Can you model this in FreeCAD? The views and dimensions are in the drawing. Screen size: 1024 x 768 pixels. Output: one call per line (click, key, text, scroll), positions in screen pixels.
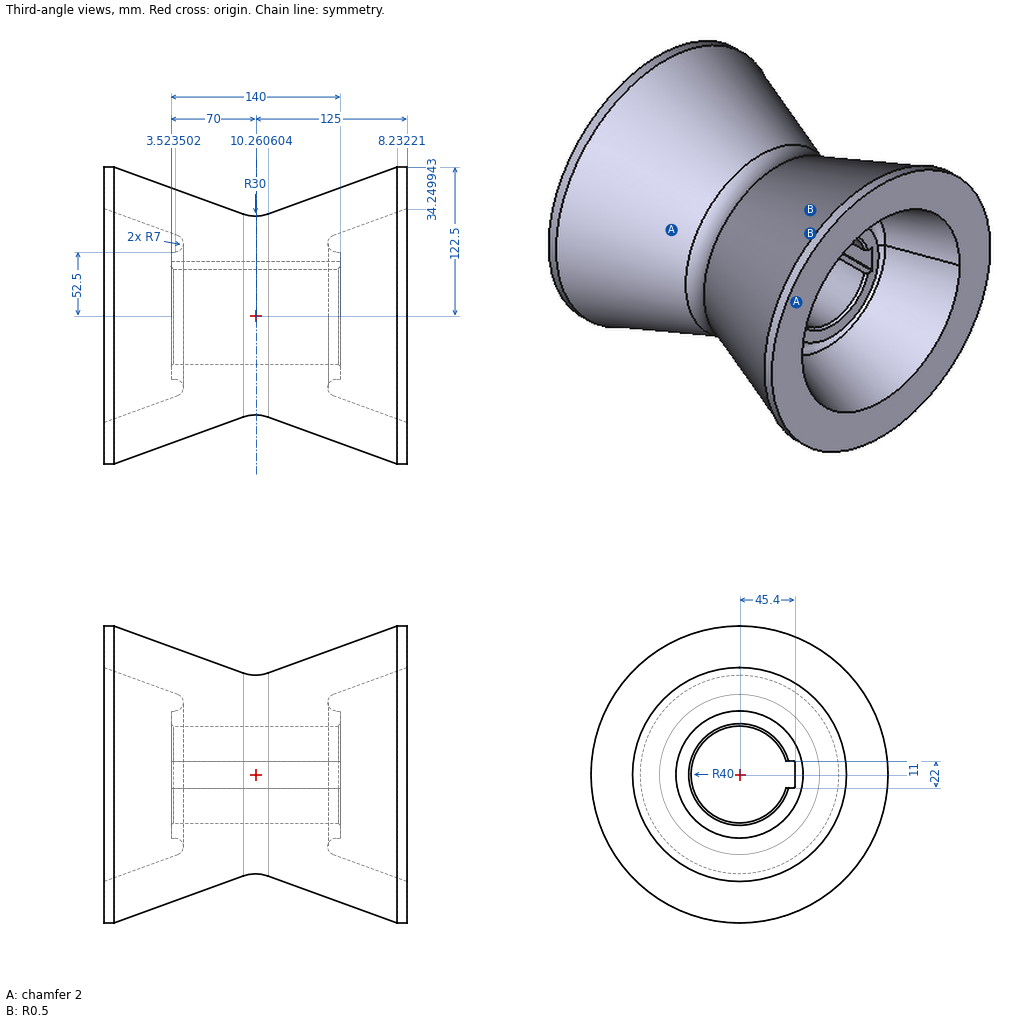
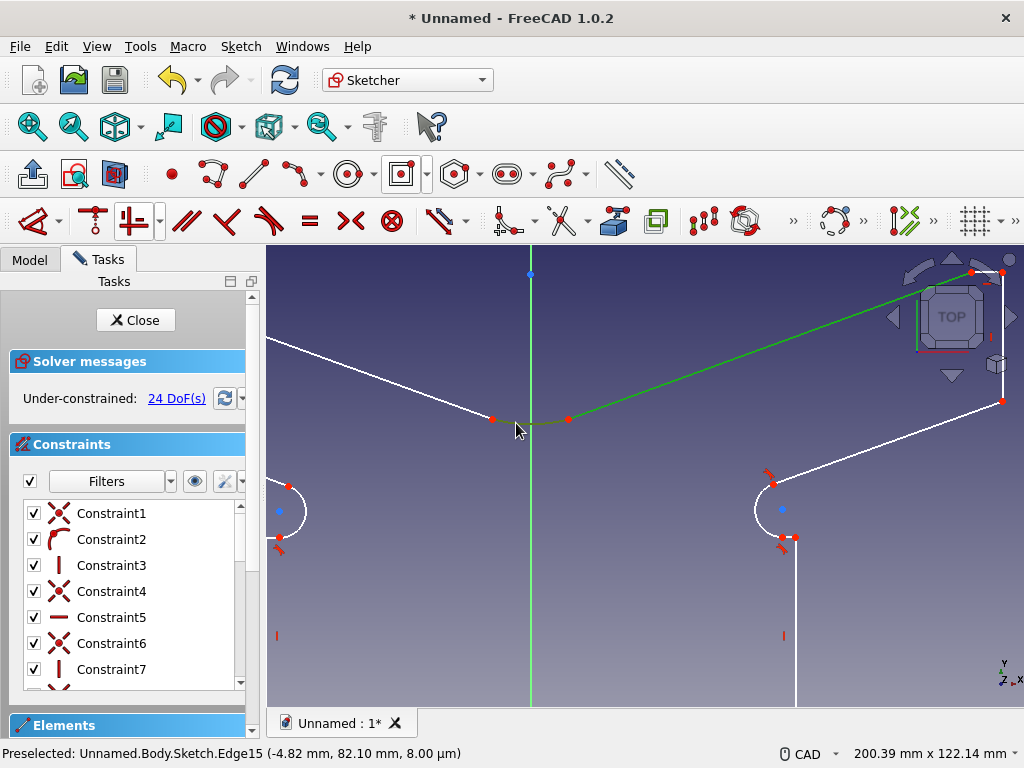
click(269, 222)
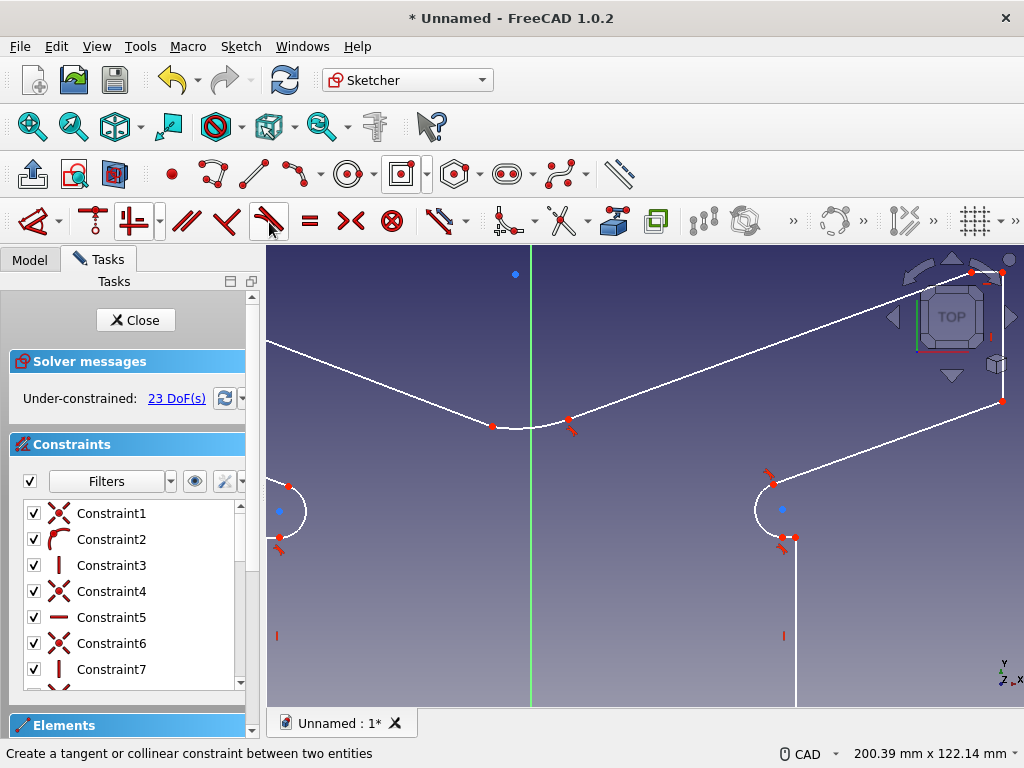
click(371, 381)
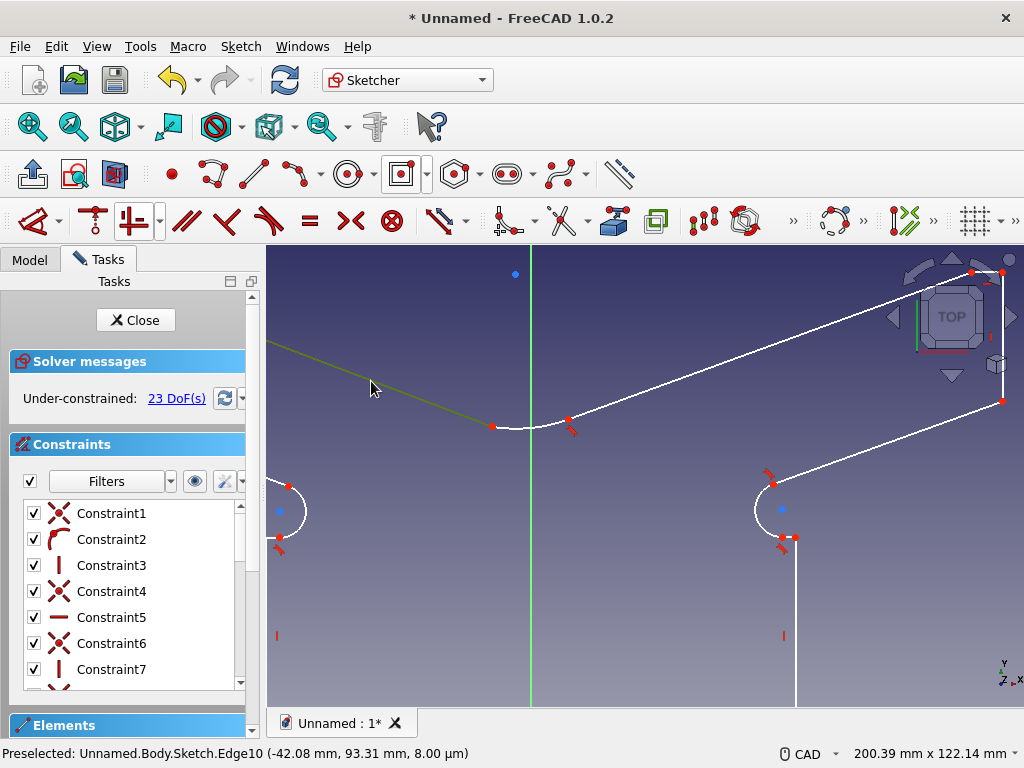
click(516, 429)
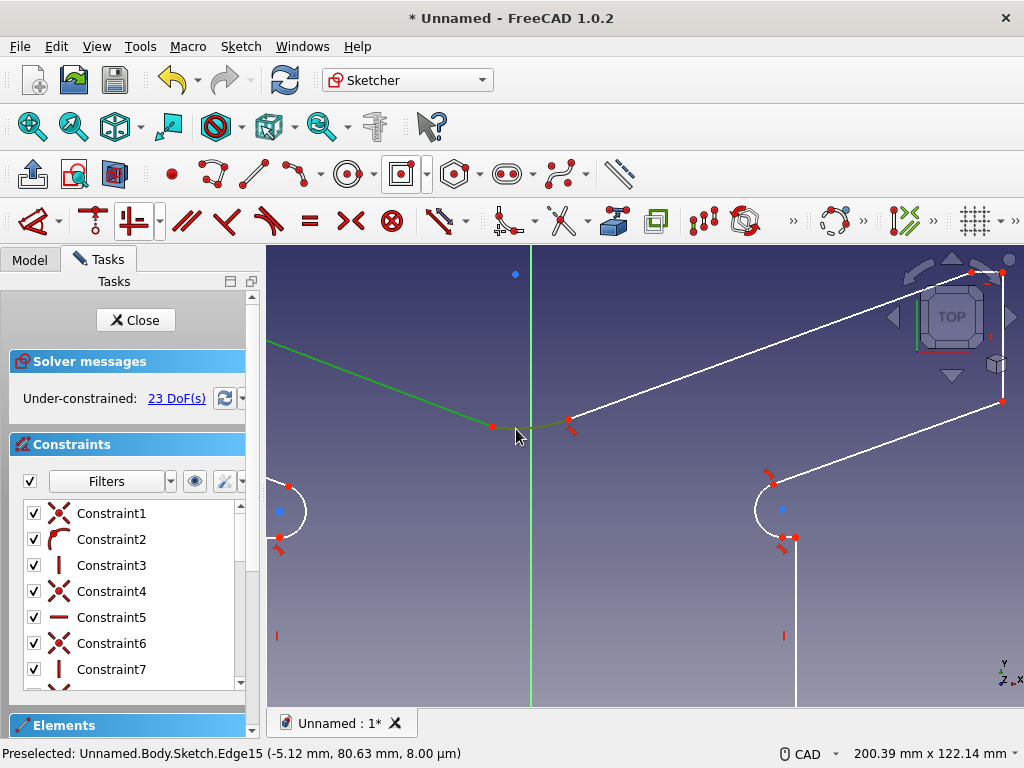
key(t)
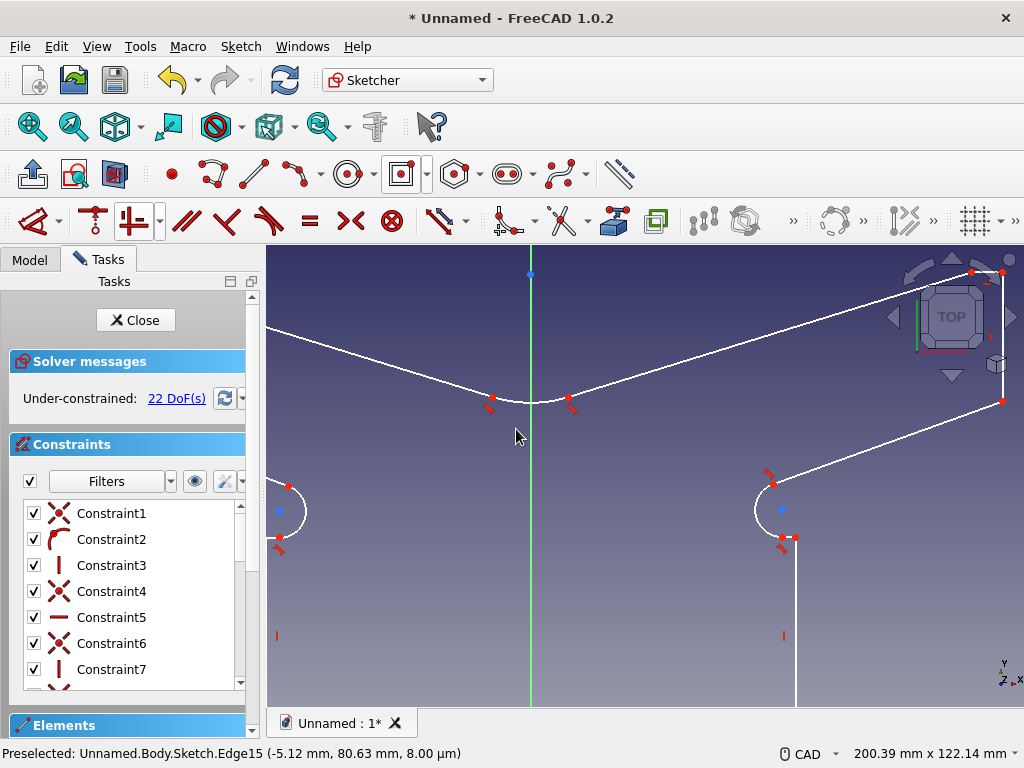
scroll(614, 455, down, 4)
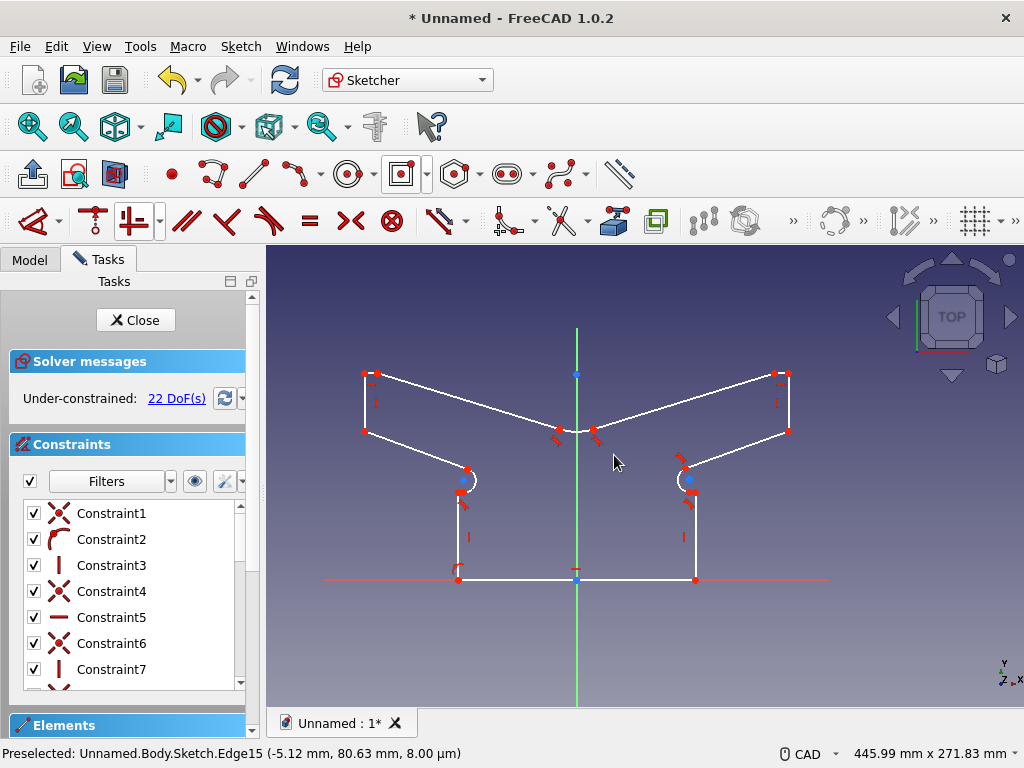
click(396, 443)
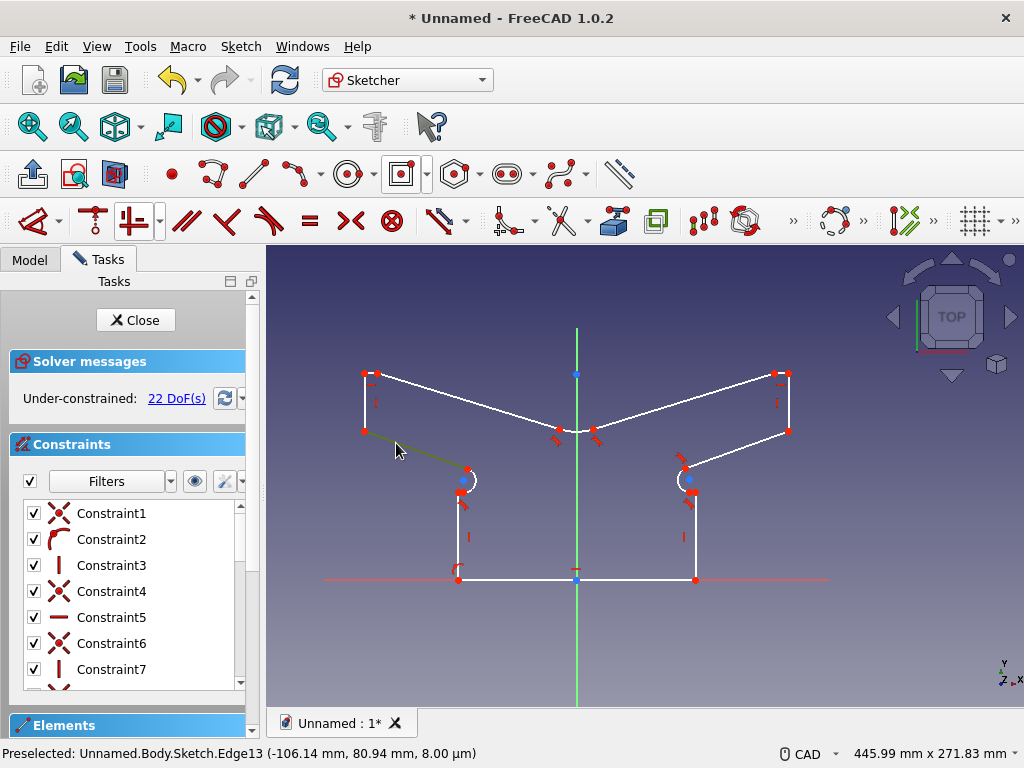
scroll(473, 489, up, 2)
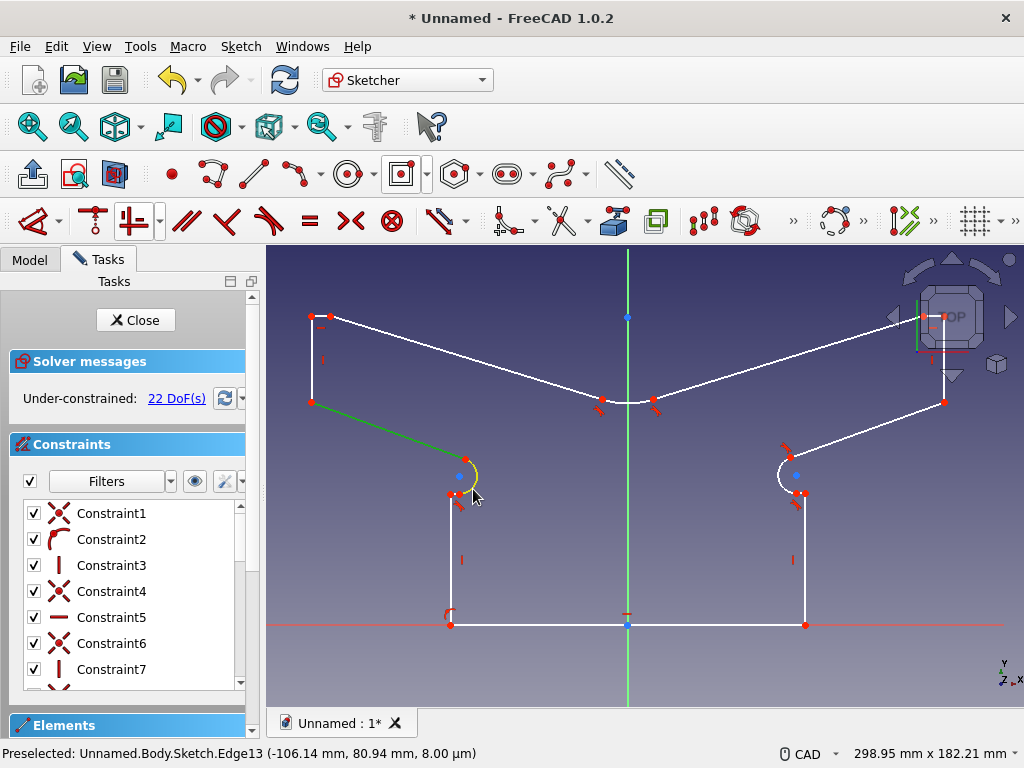
click(473, 488)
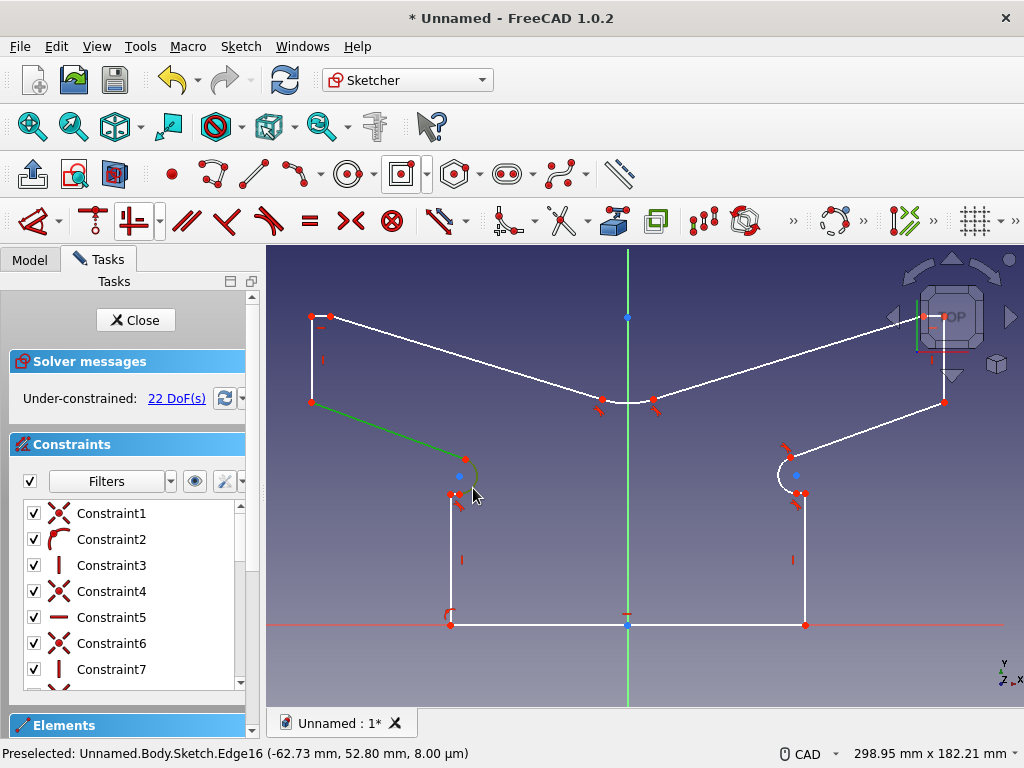
click(269, 222)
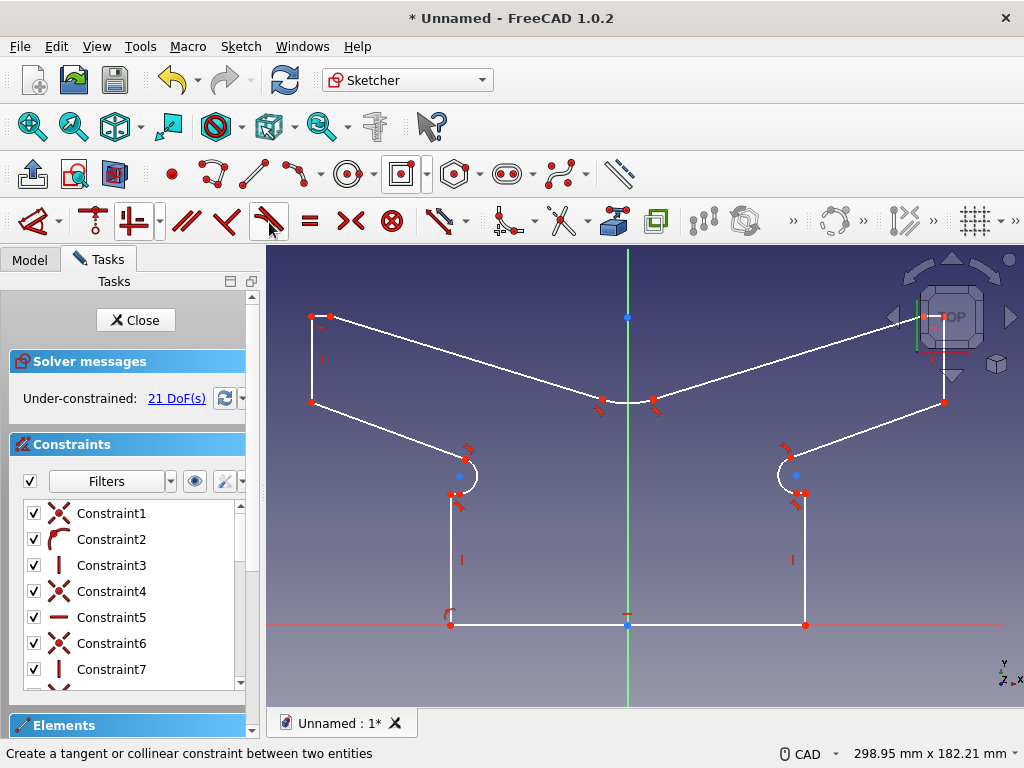
scroll(455, 494, up, 6)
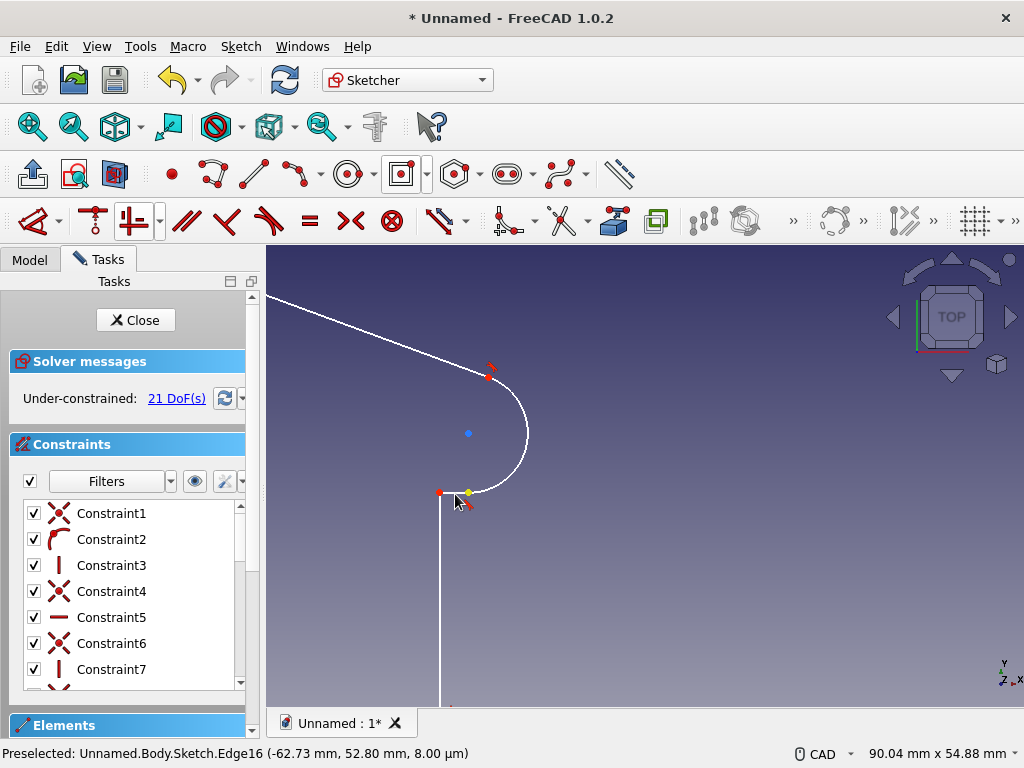
click(454, 493)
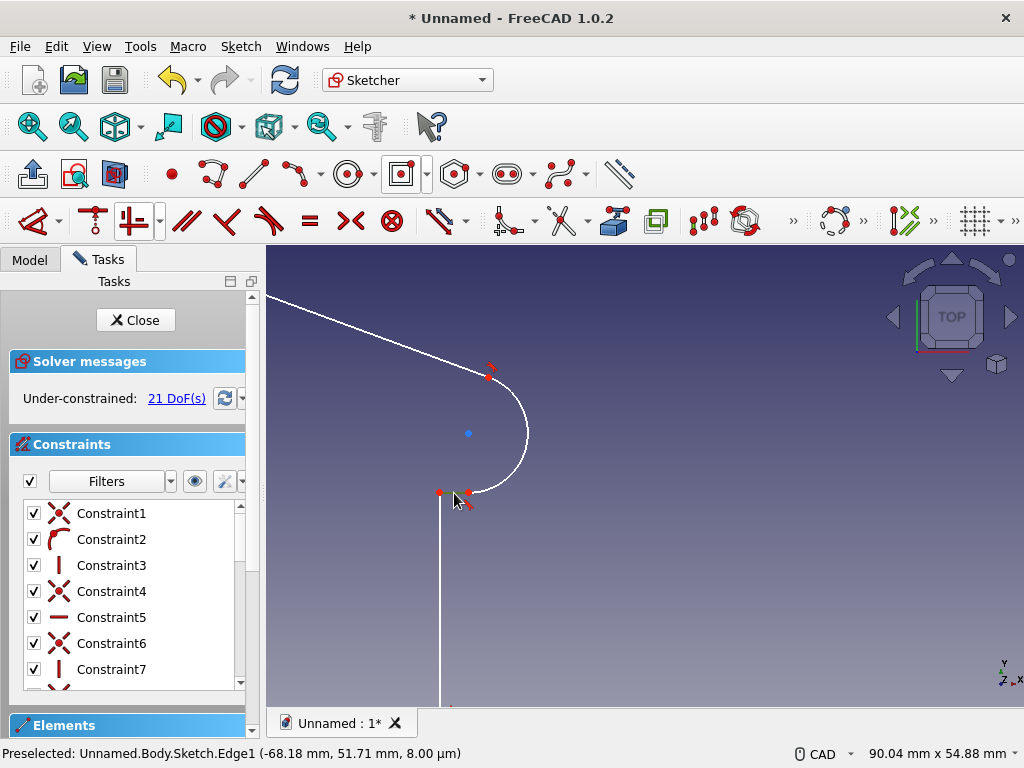
key(h)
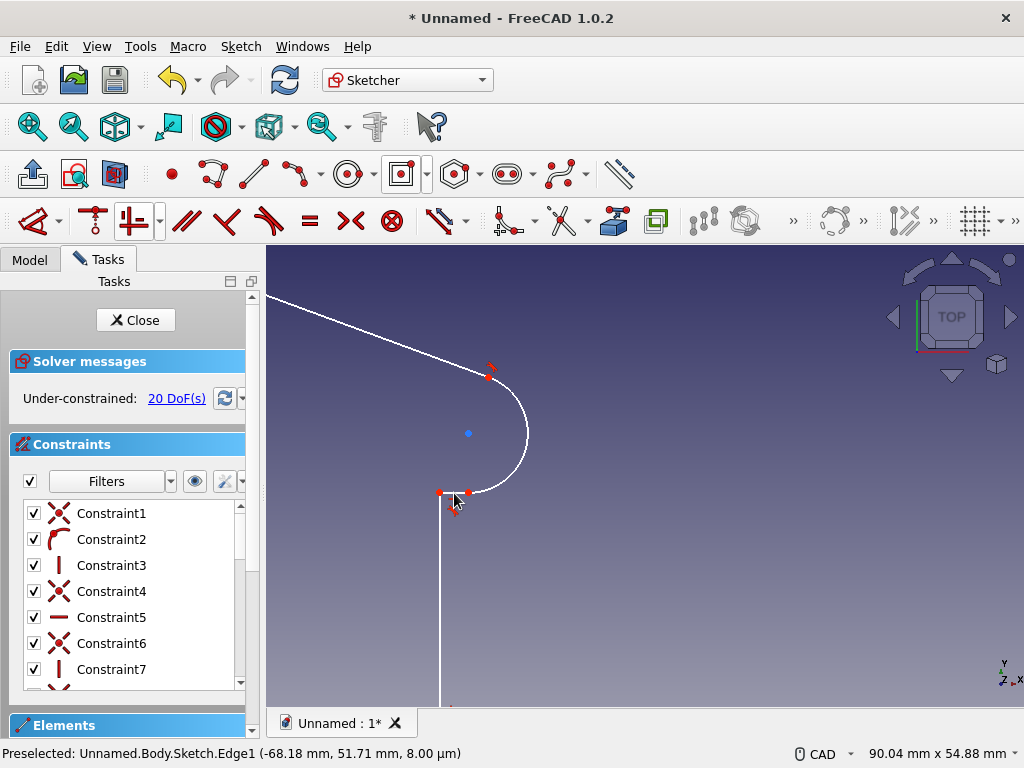
scroll(462, 492, down, 8)